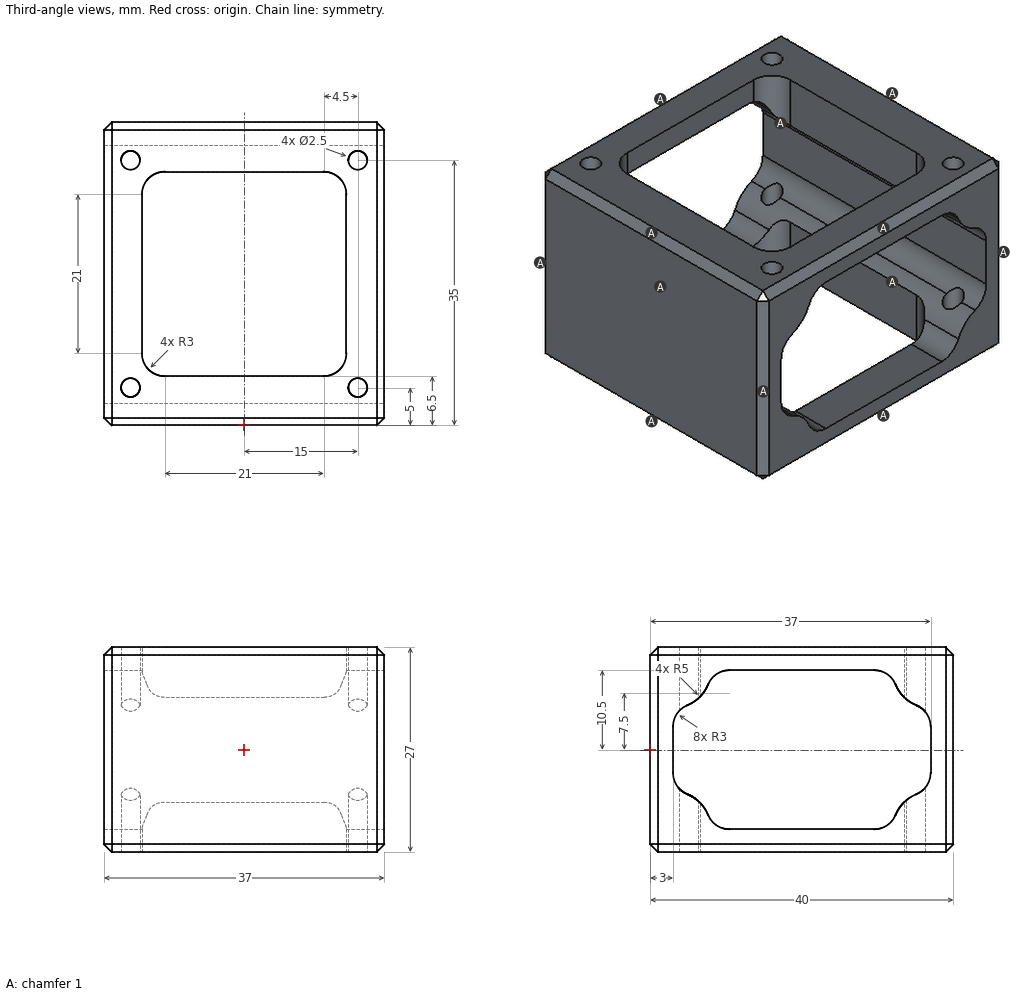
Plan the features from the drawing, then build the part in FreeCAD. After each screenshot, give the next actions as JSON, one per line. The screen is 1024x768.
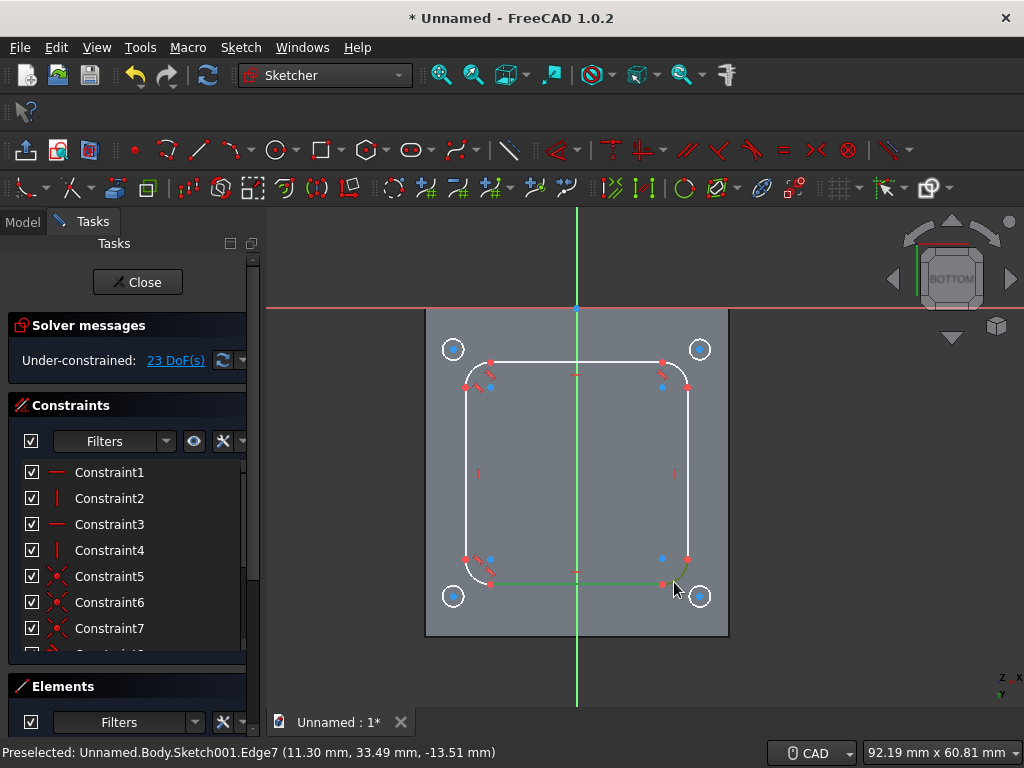
{"action": "key", "text": "t"}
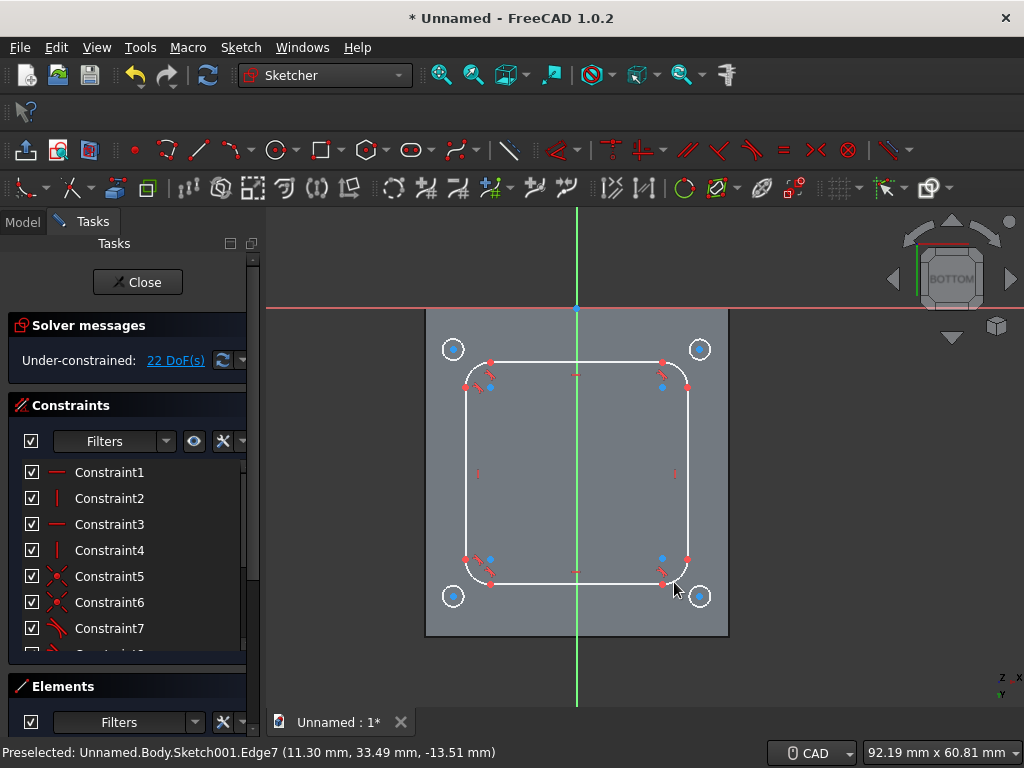
{"action": "left_click", "coordinate": [688, 508]}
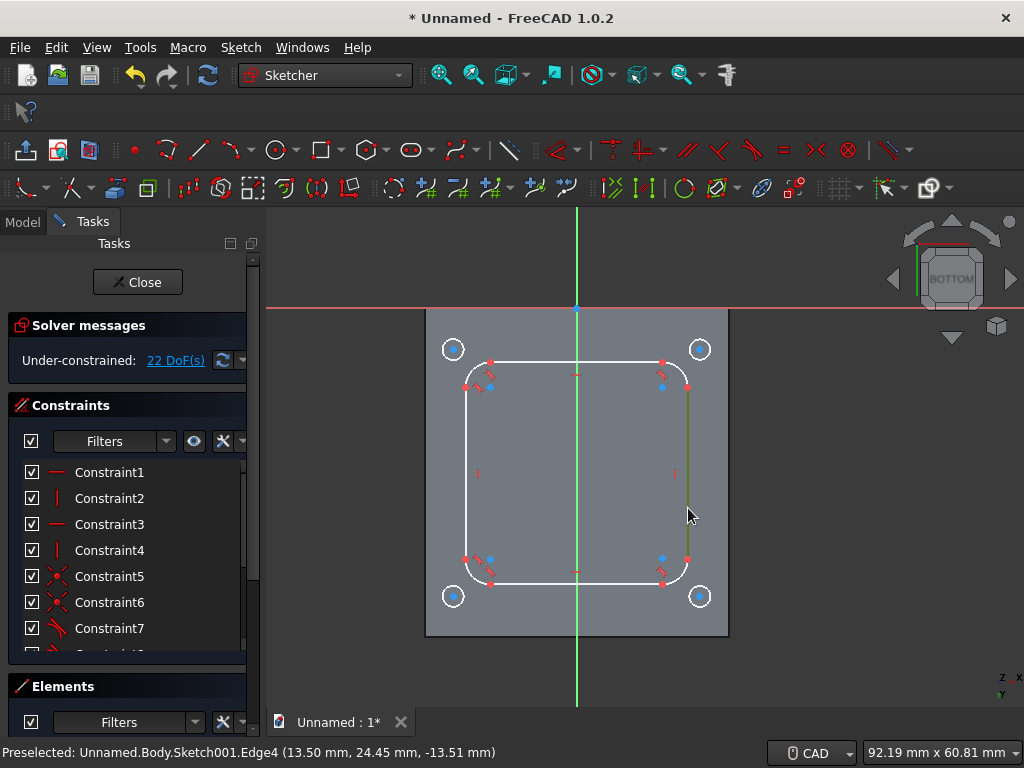
{"action": "left_click", "coordinate": [674, 582]}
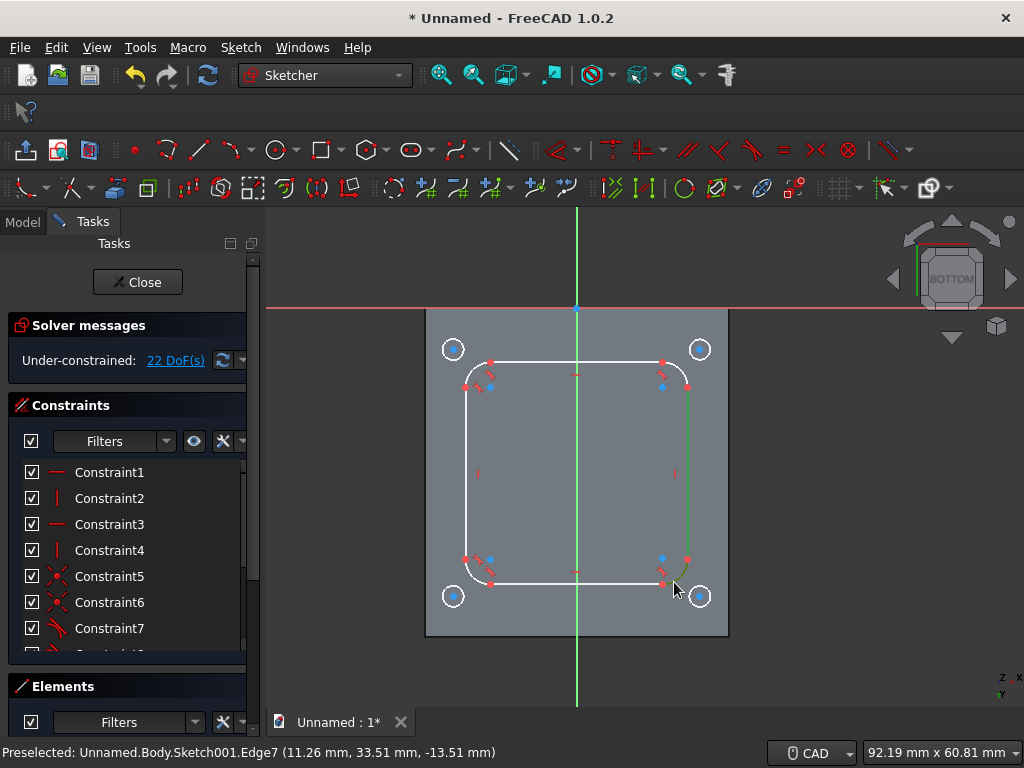
{"action": "key", "text": "t"}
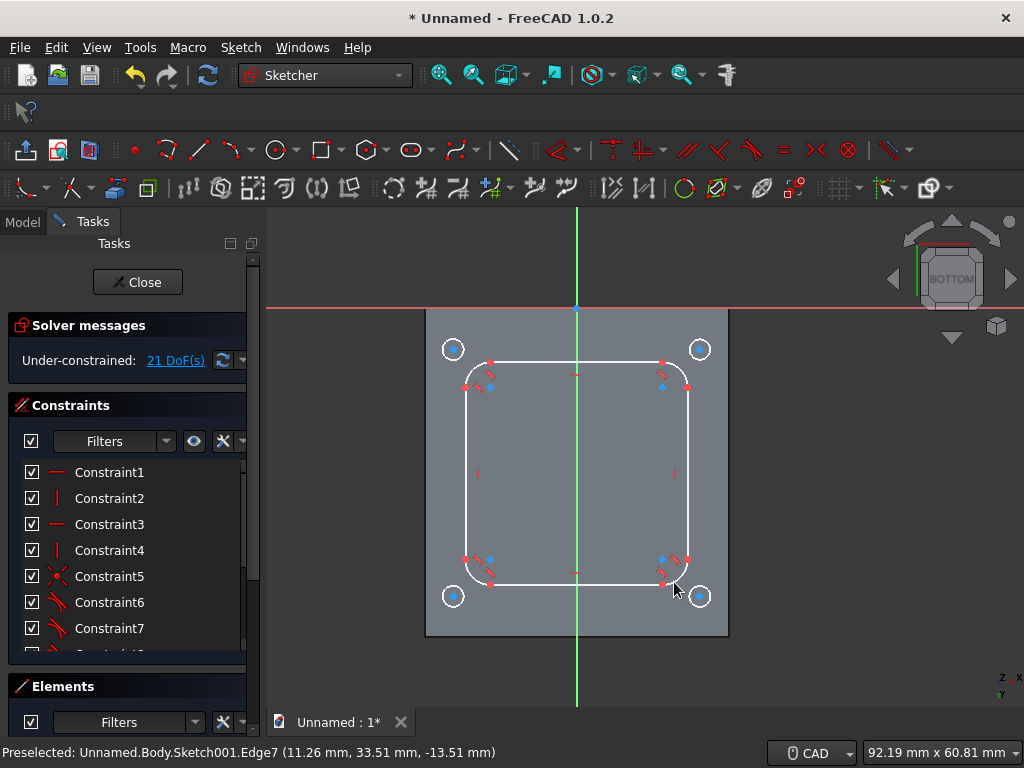
{"action": "left_click", "coordinate": [688, 508]}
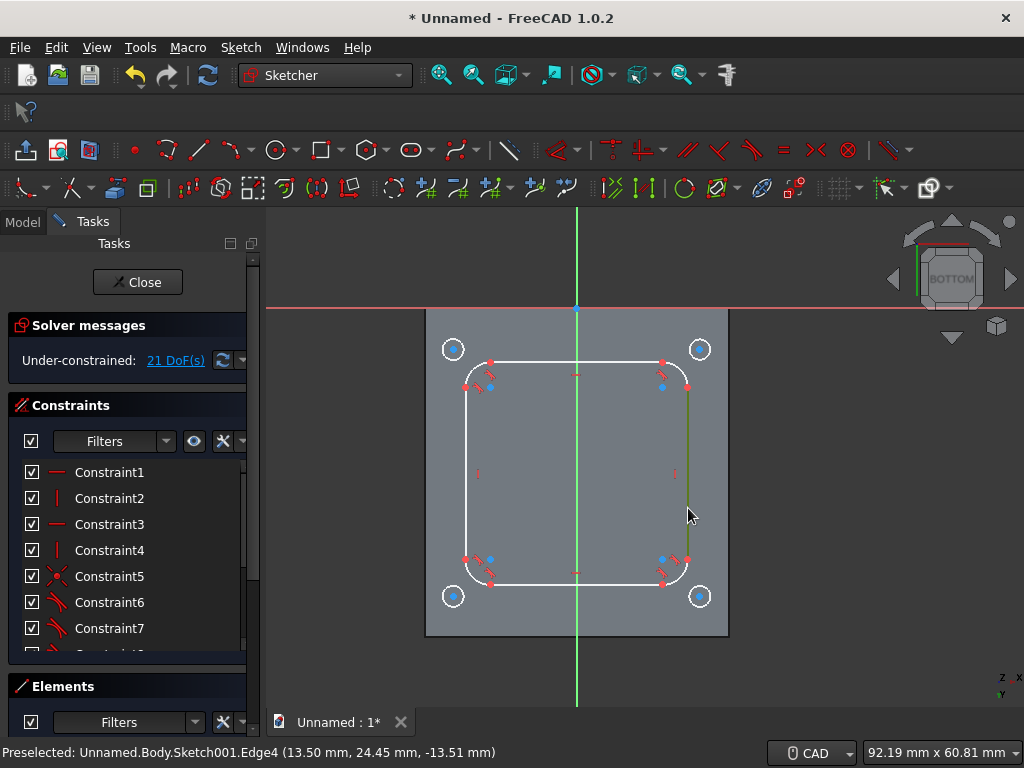
{"action": "left_click", "coordinate": [685, 376]}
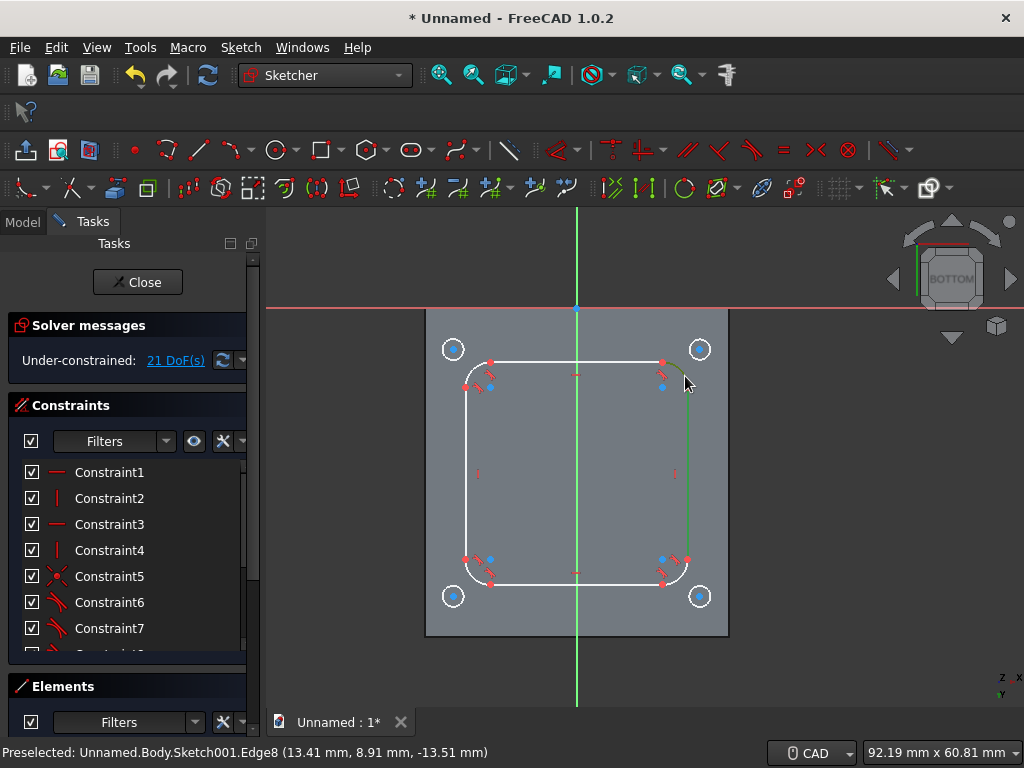
{"action": "left_click", "coordinate": [752, 150]}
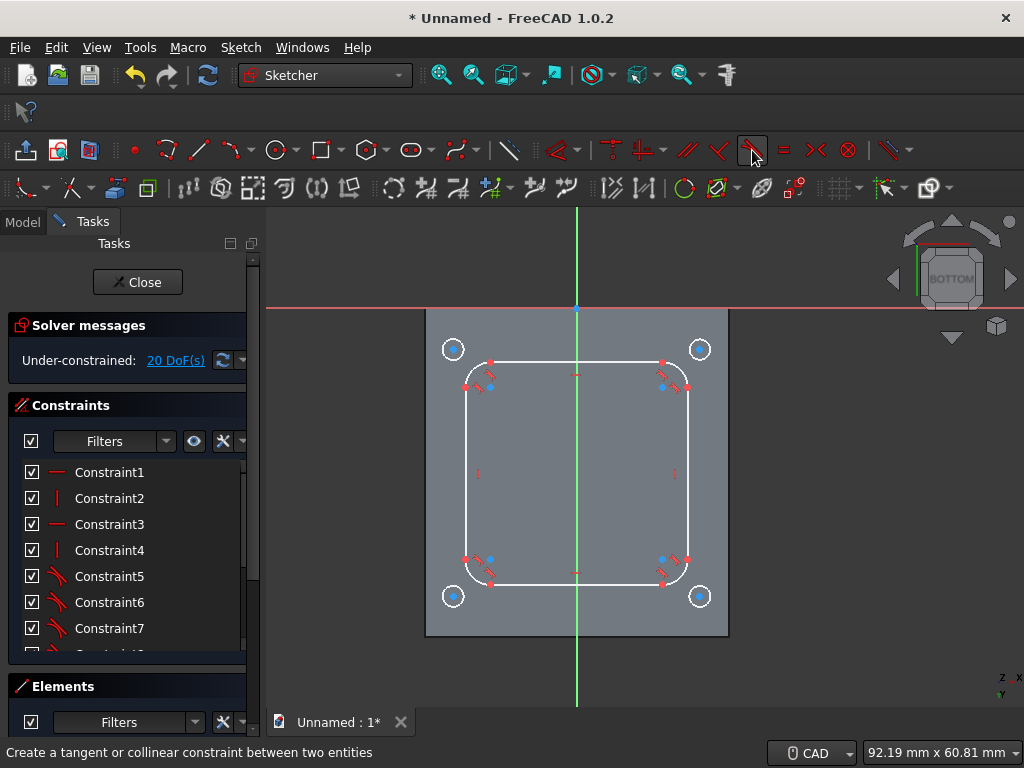
{"action": "left_click", "coordinate": [479, 365]}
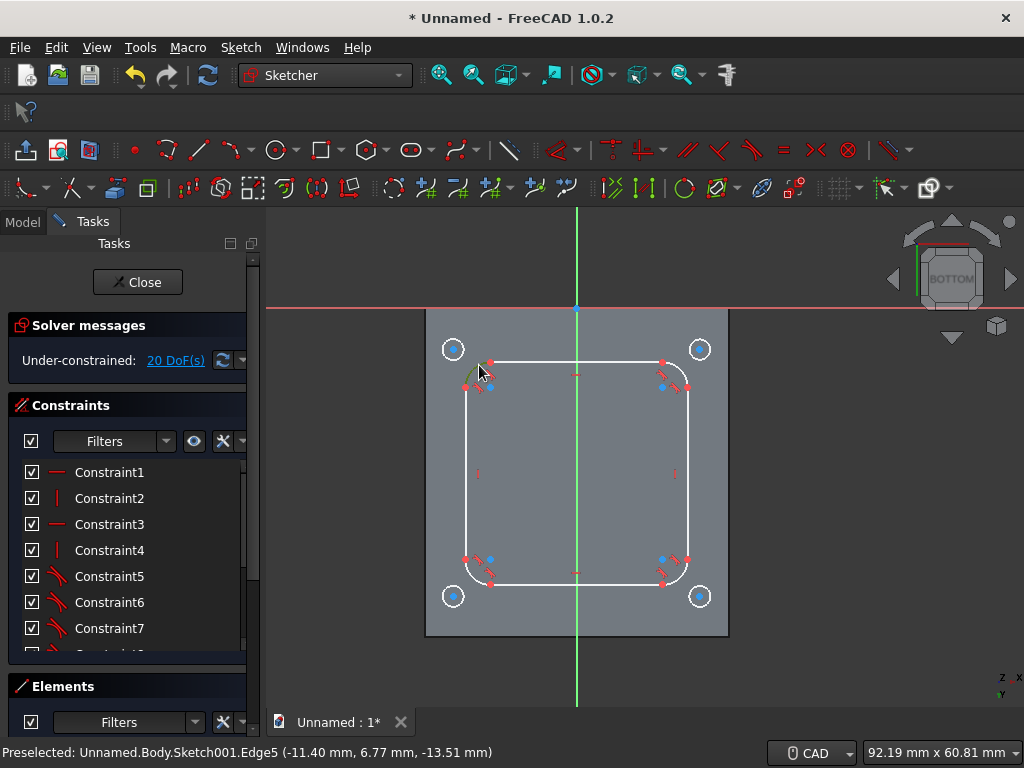
{"action": "left_click", "coordinate": [468, 571]}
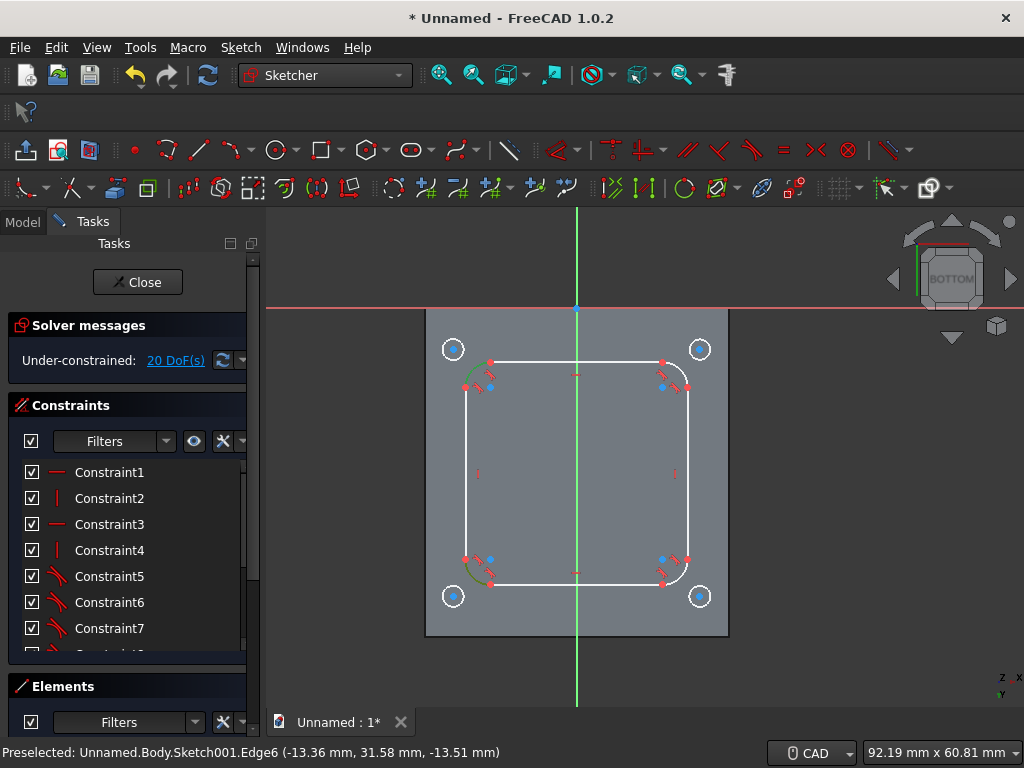
{"action": "left_click", "coordinate": [674, 582]}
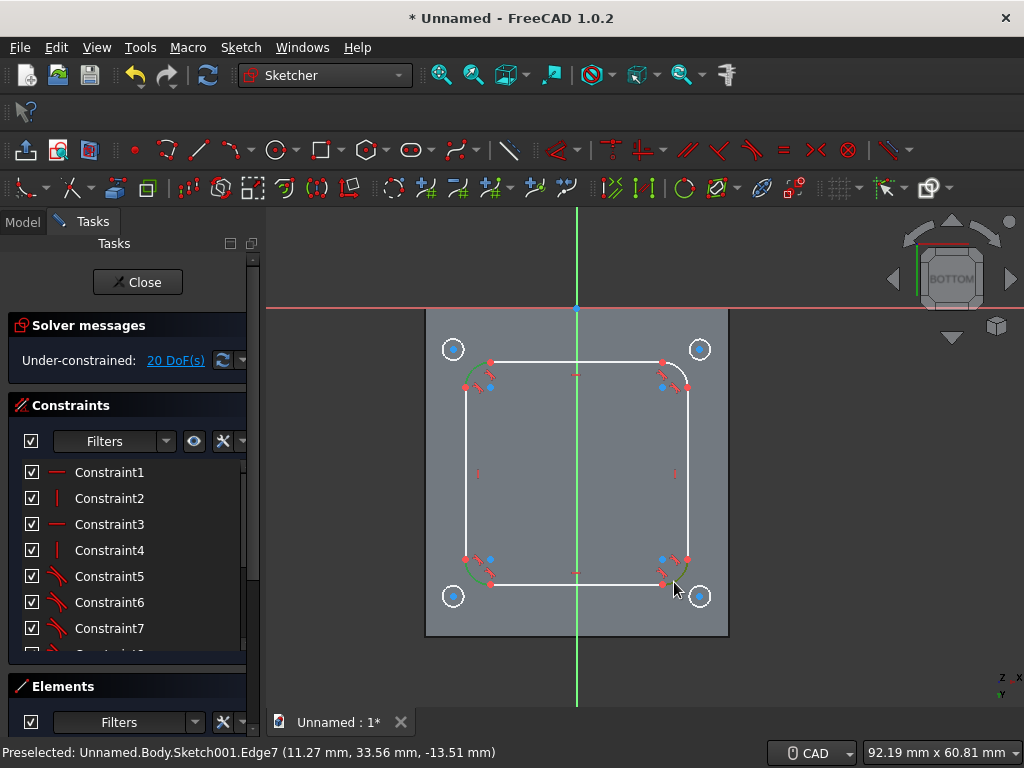
{"action": "left_click", "coordinate": [685, 376]}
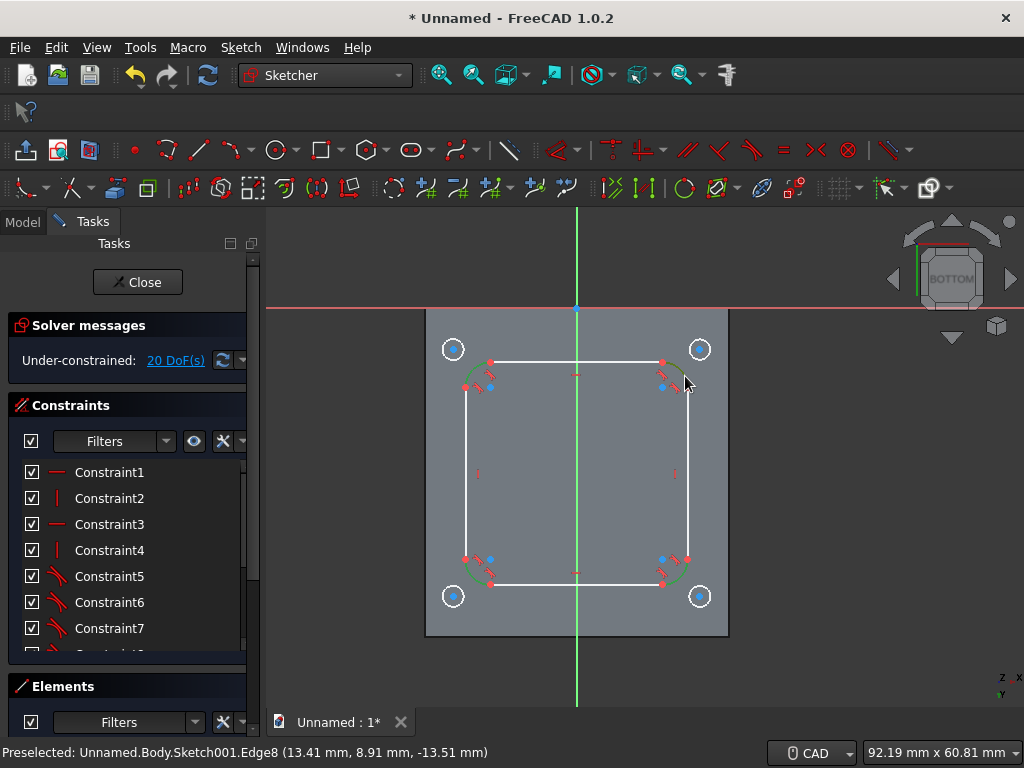
{"action": "key", "text": "e"}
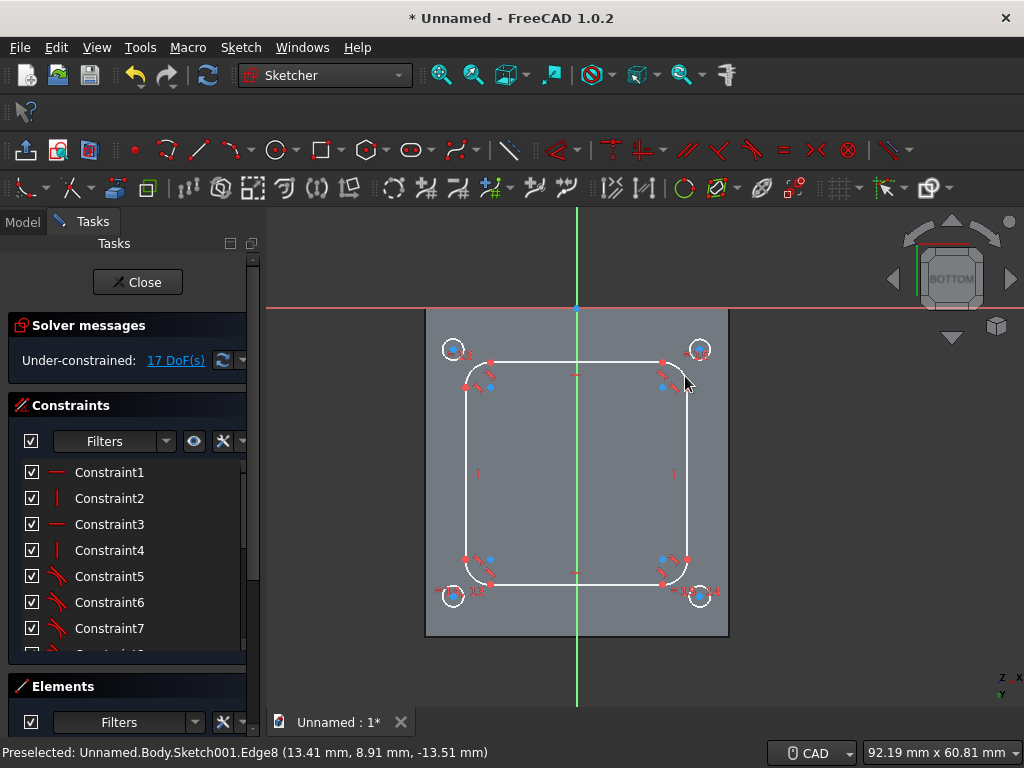
{"action": "scroll", "coordinate": [707, 589], "scroll_direction": "up", "scroll_amount": 2}